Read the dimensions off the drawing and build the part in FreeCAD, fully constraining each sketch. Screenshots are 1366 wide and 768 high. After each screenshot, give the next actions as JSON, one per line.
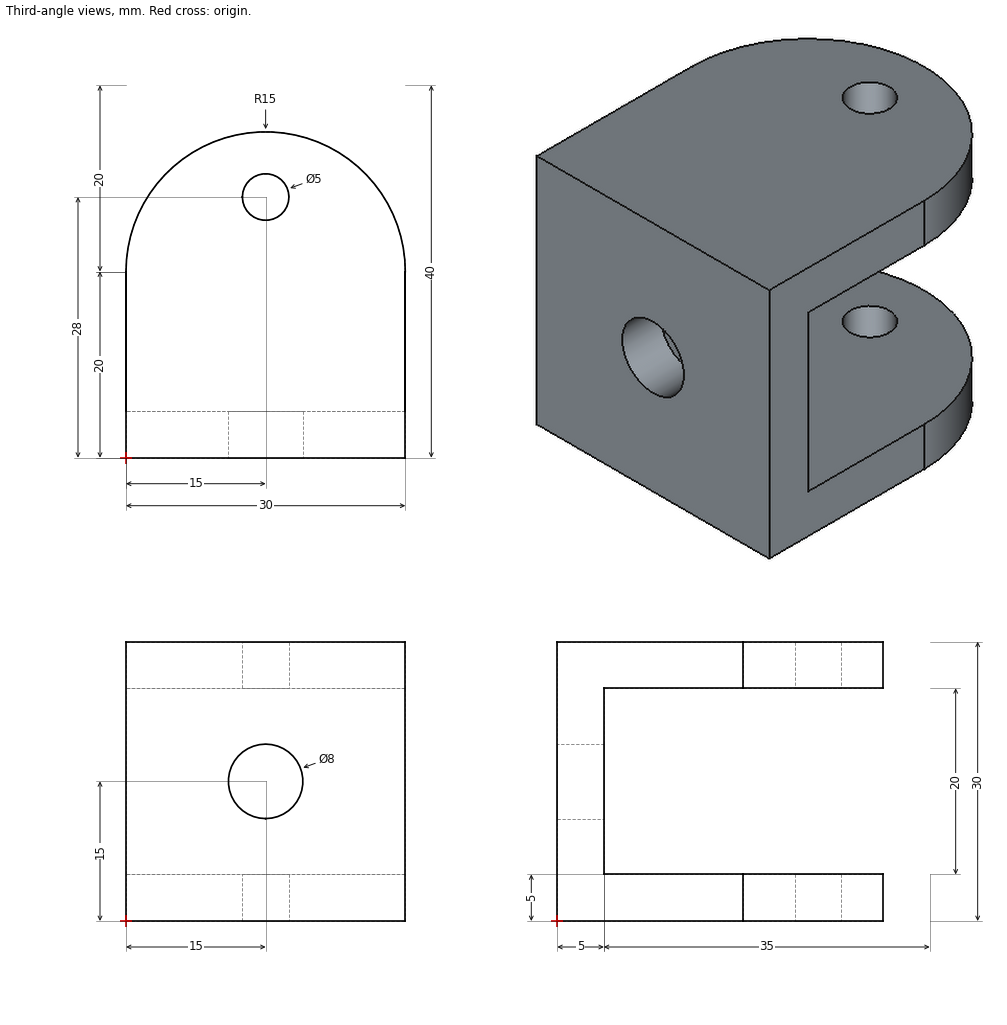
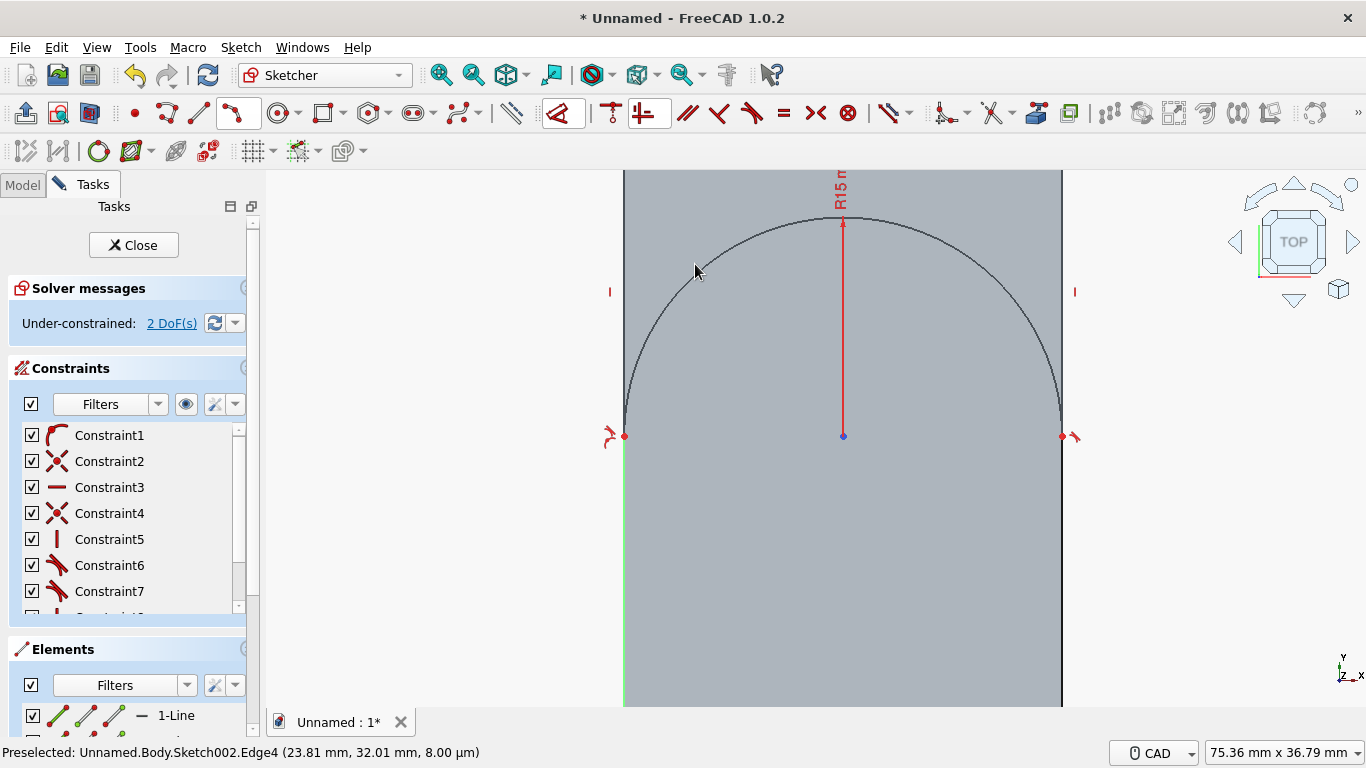
{"action": "left_click", "coordinate": [624, 349]}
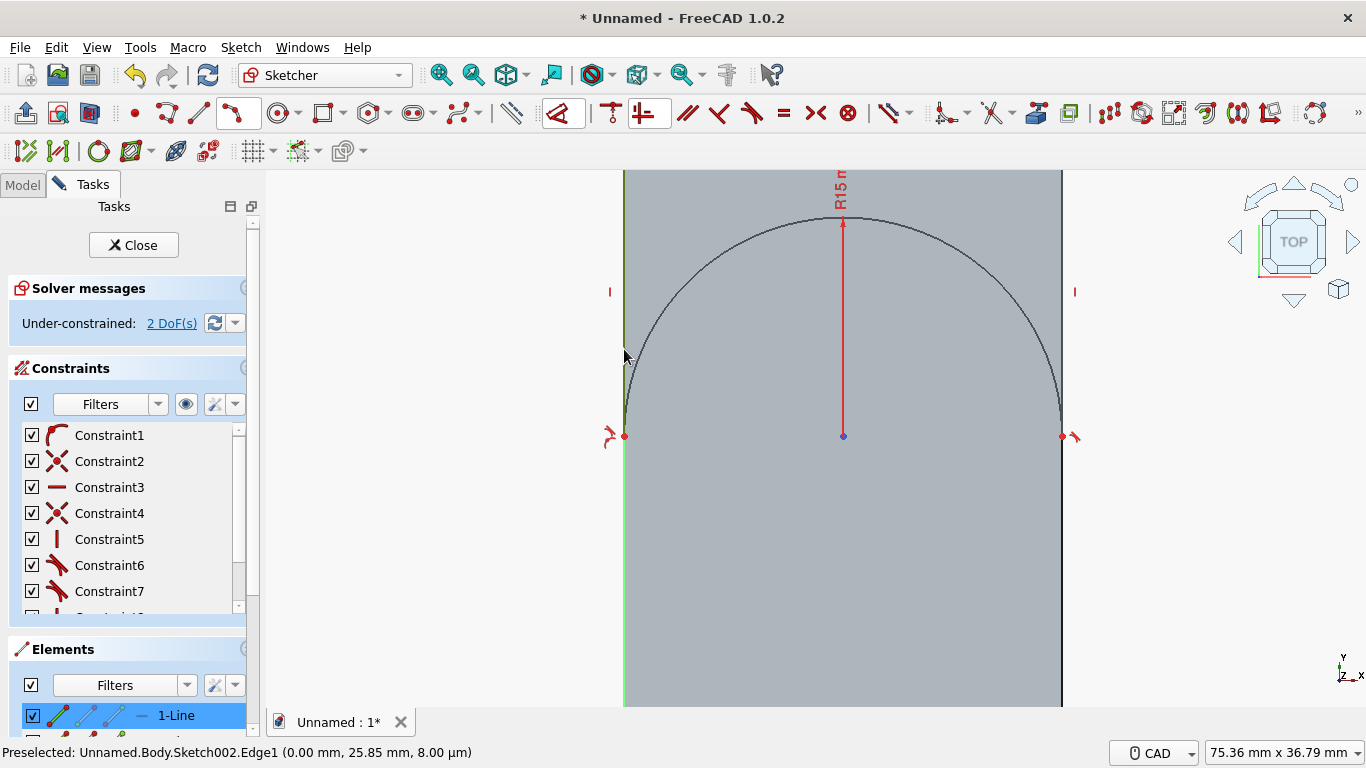
{"action": "key", "text": "i"}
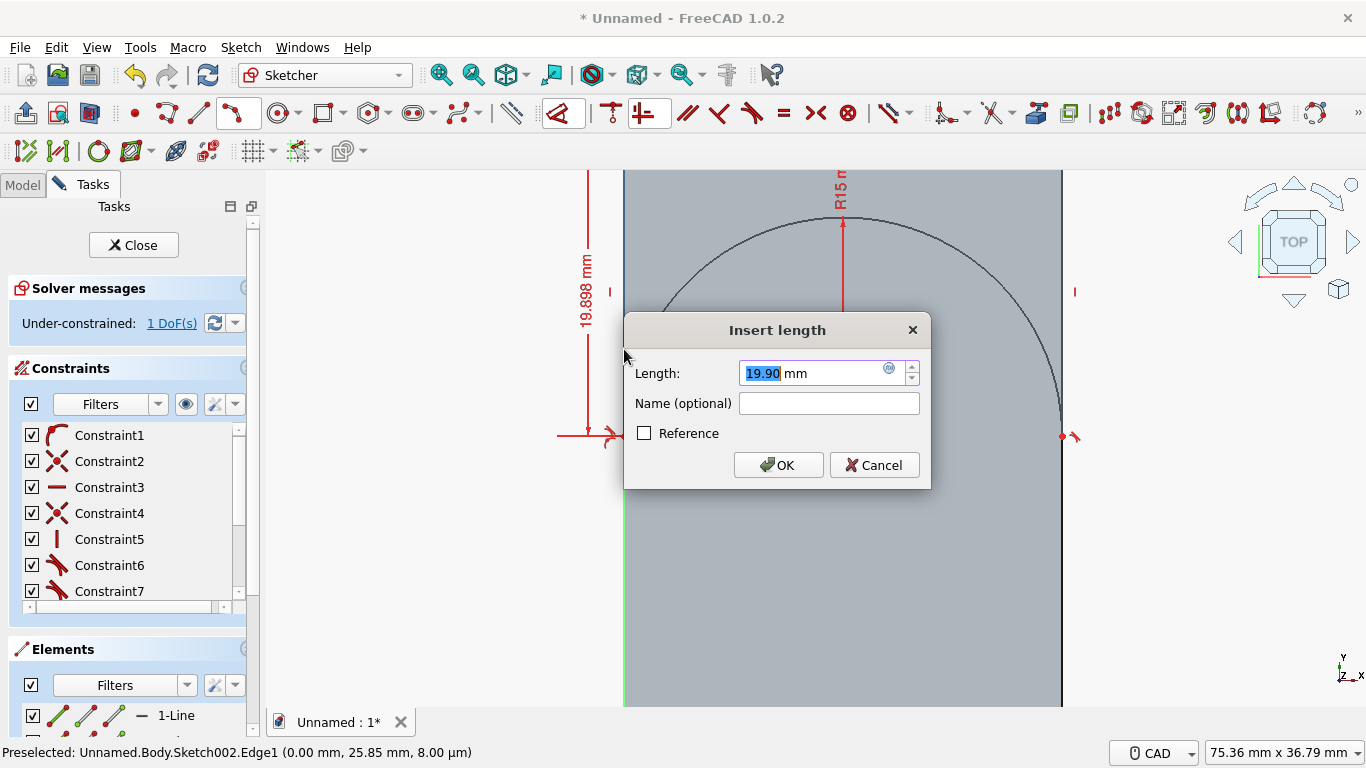
{"action": "type", "text": "20"}
{"action": "key", "text": "Return"}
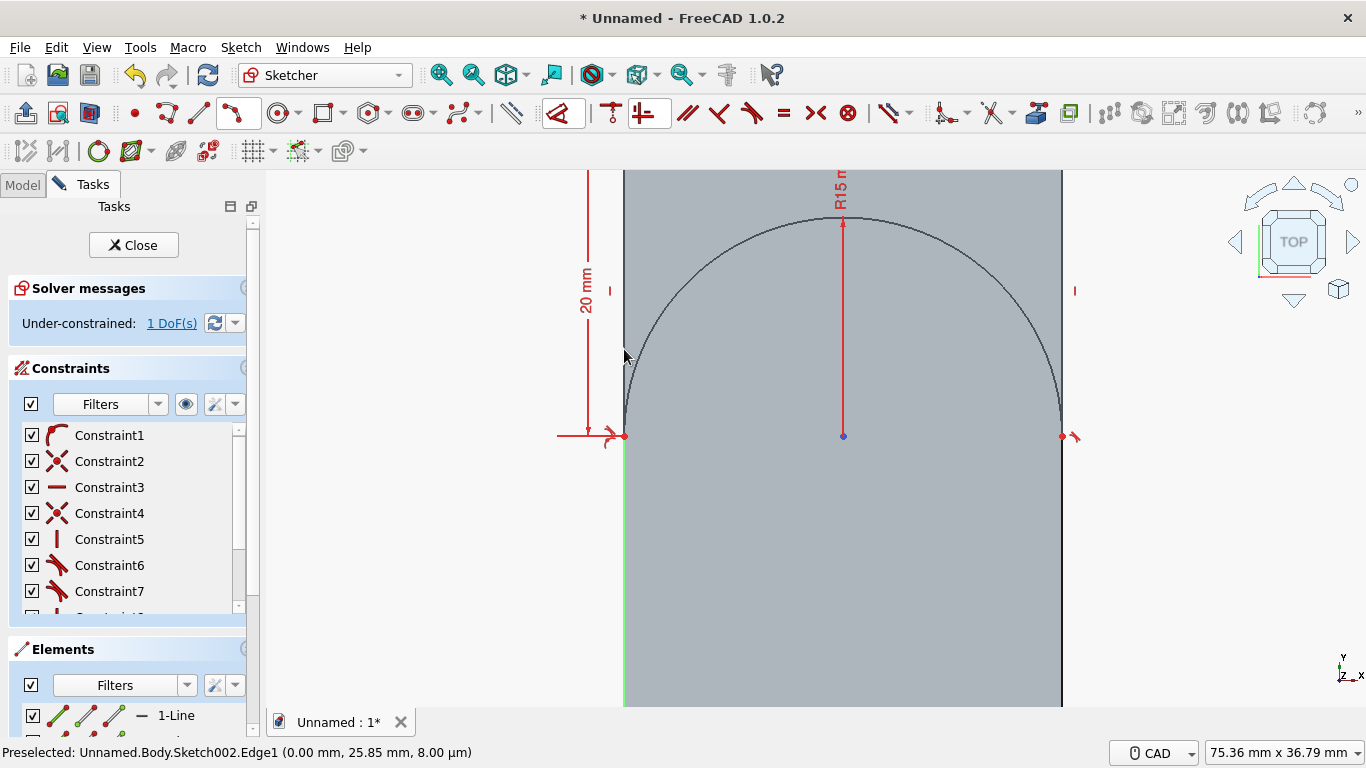
{"action": "left_click", "coordinate": [624, 436]}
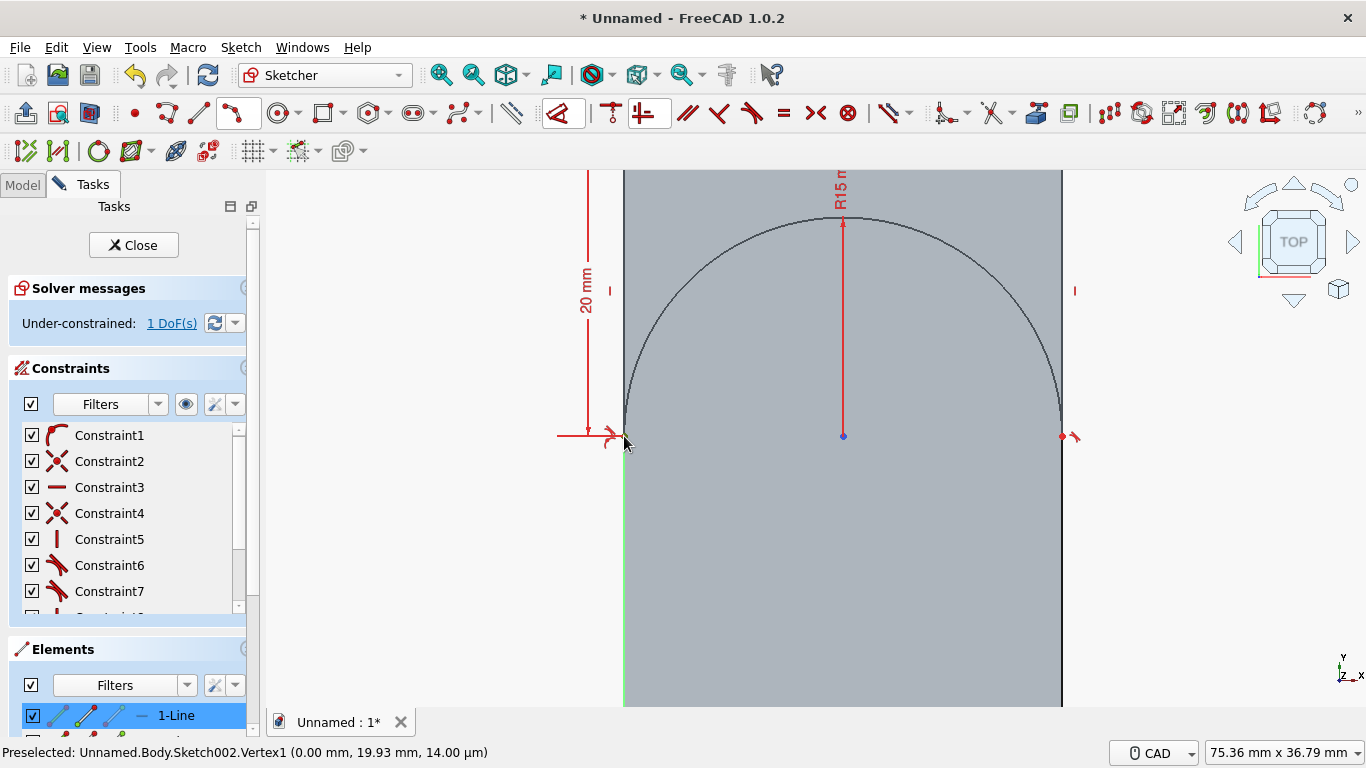
{"action": "left_click", "coordinate": [580, 114]}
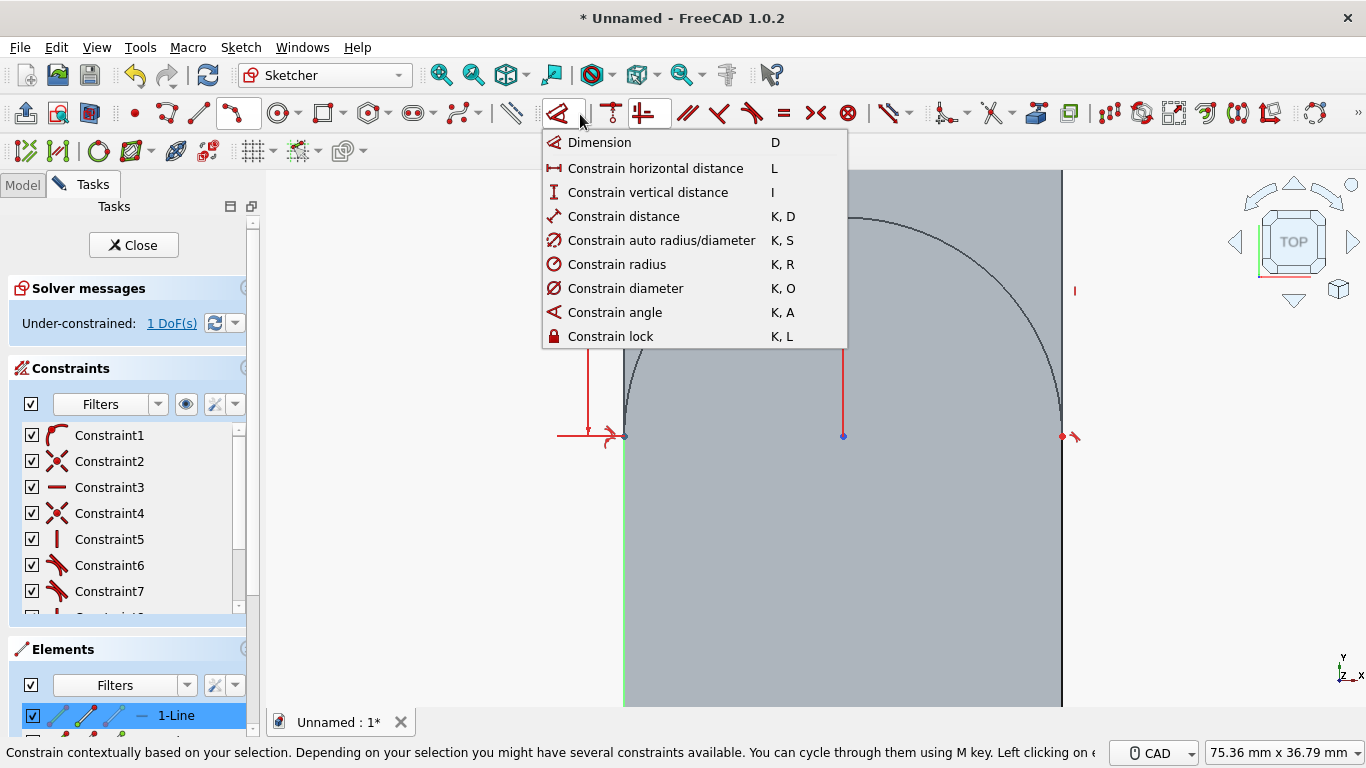
{"action": "left_click", "coordinate": [695, 192]}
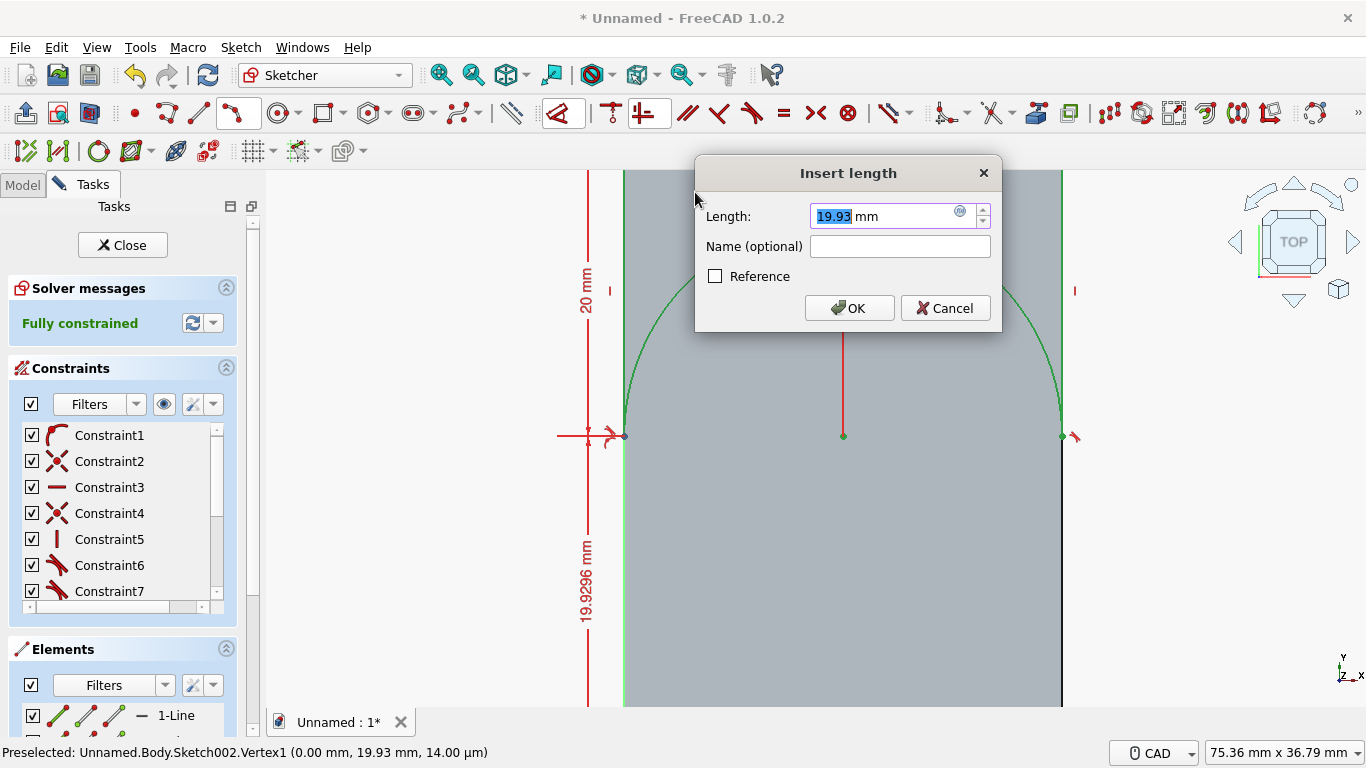
{"action": "type", "text": "20"}
{"action": "key", "text": "Return"}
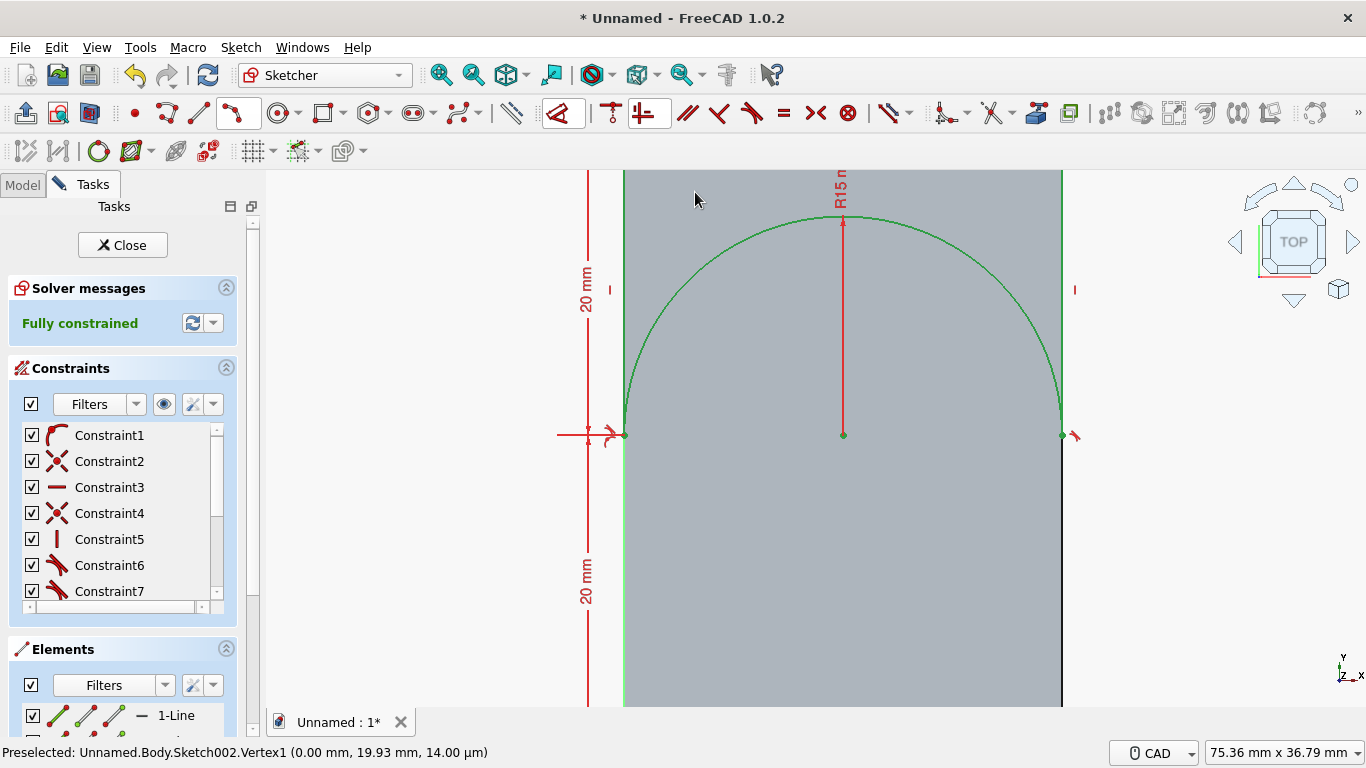
{"action": "left_click", "coordinate": [123, 245]}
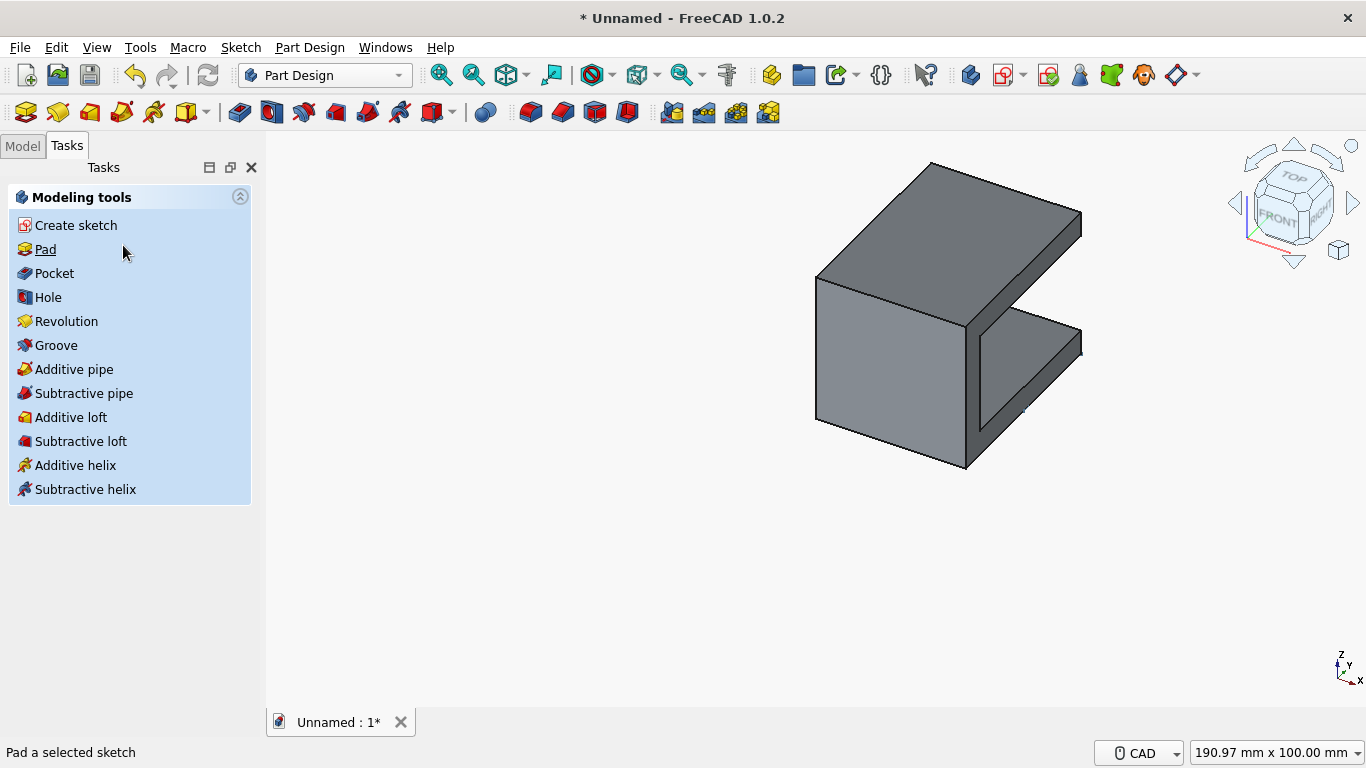
{"action": "left_click", "coordinate": [240, 112]}